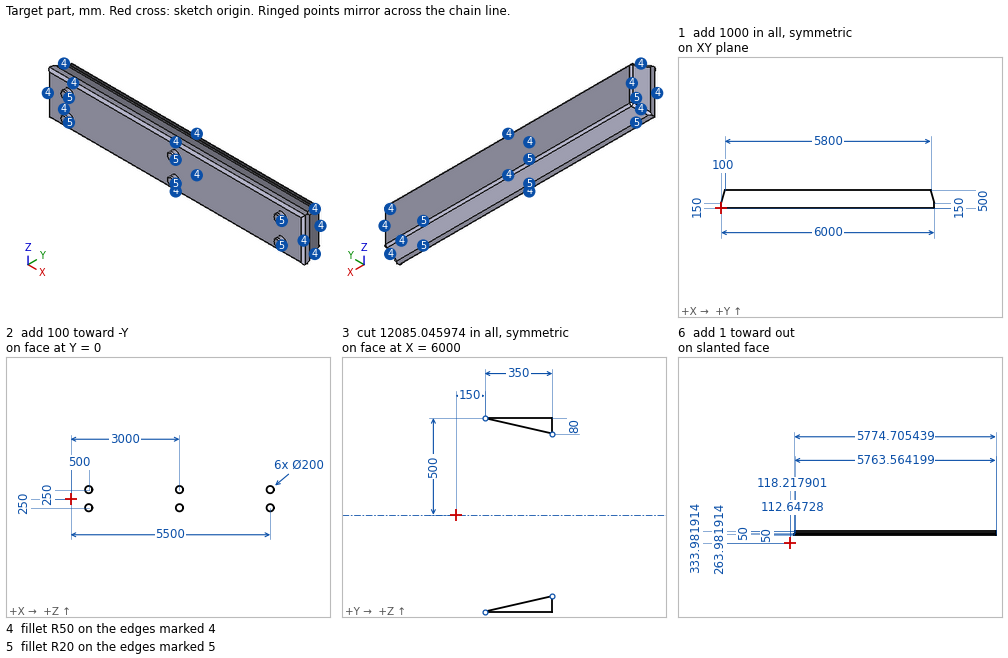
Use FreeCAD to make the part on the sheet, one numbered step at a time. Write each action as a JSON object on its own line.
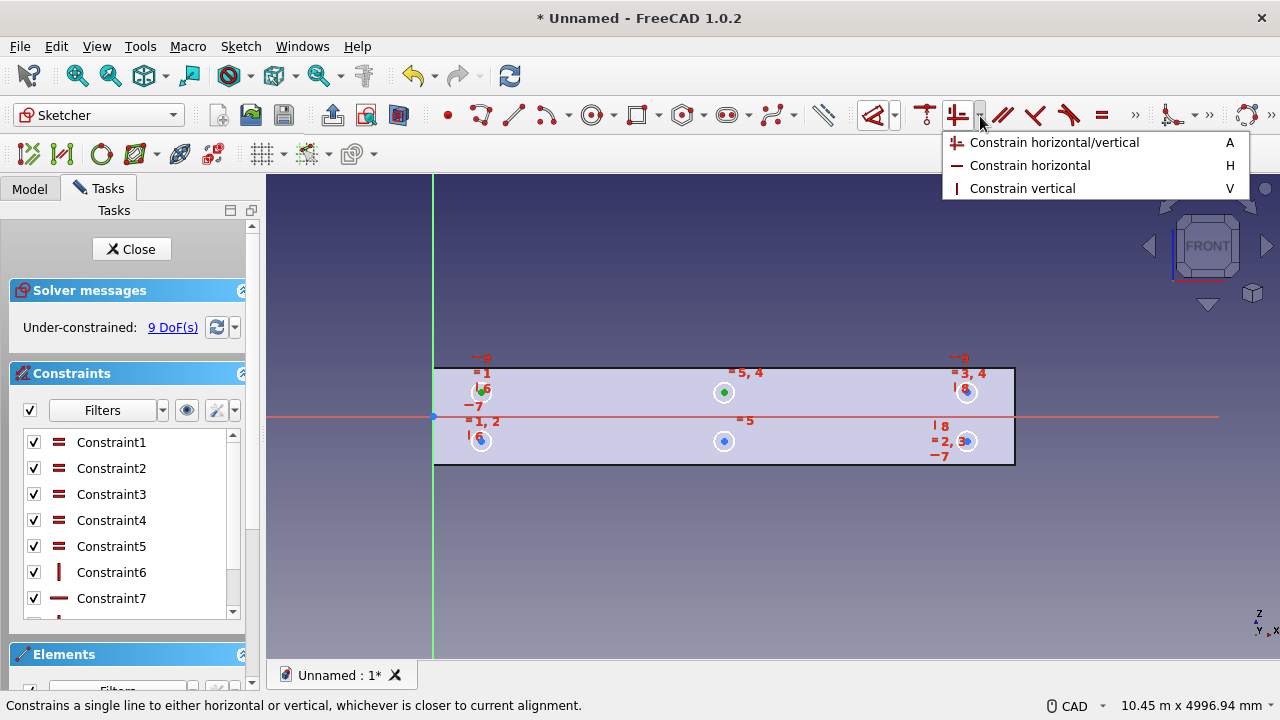
{"action": "left_click", "coordinate": [1096, 166]}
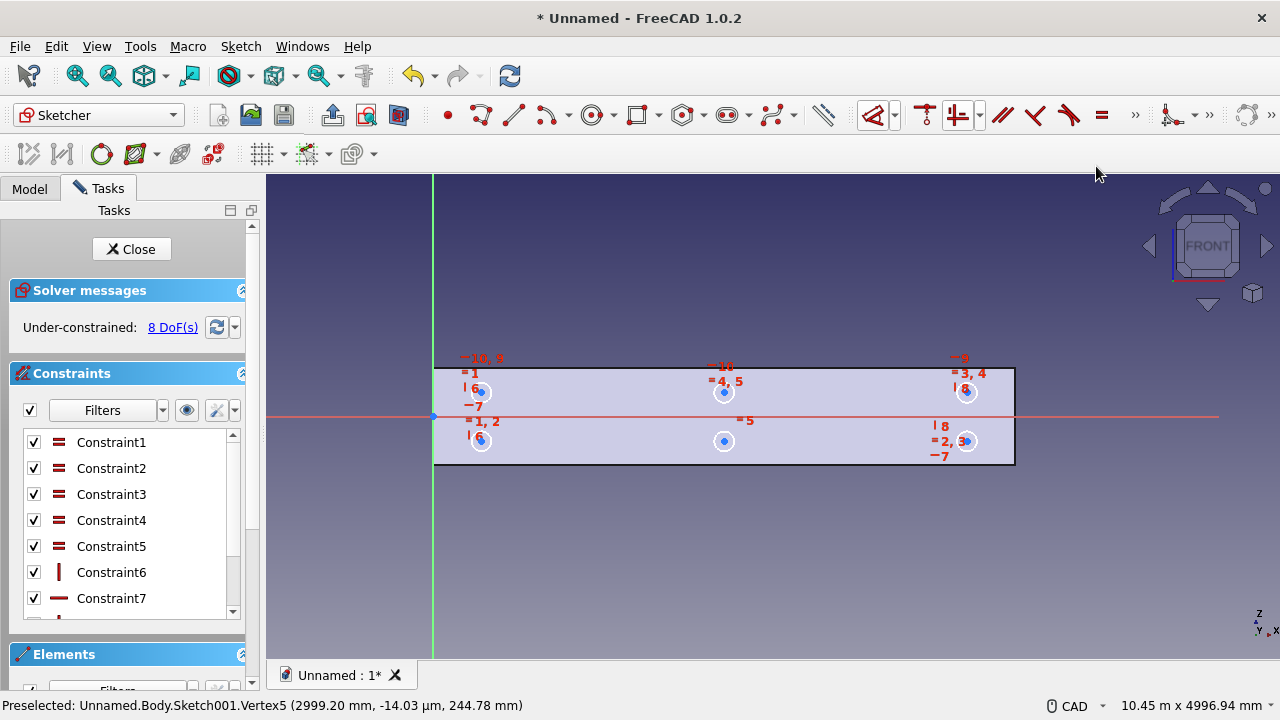
{"action": "left_click", "coordinate": [724, 393]}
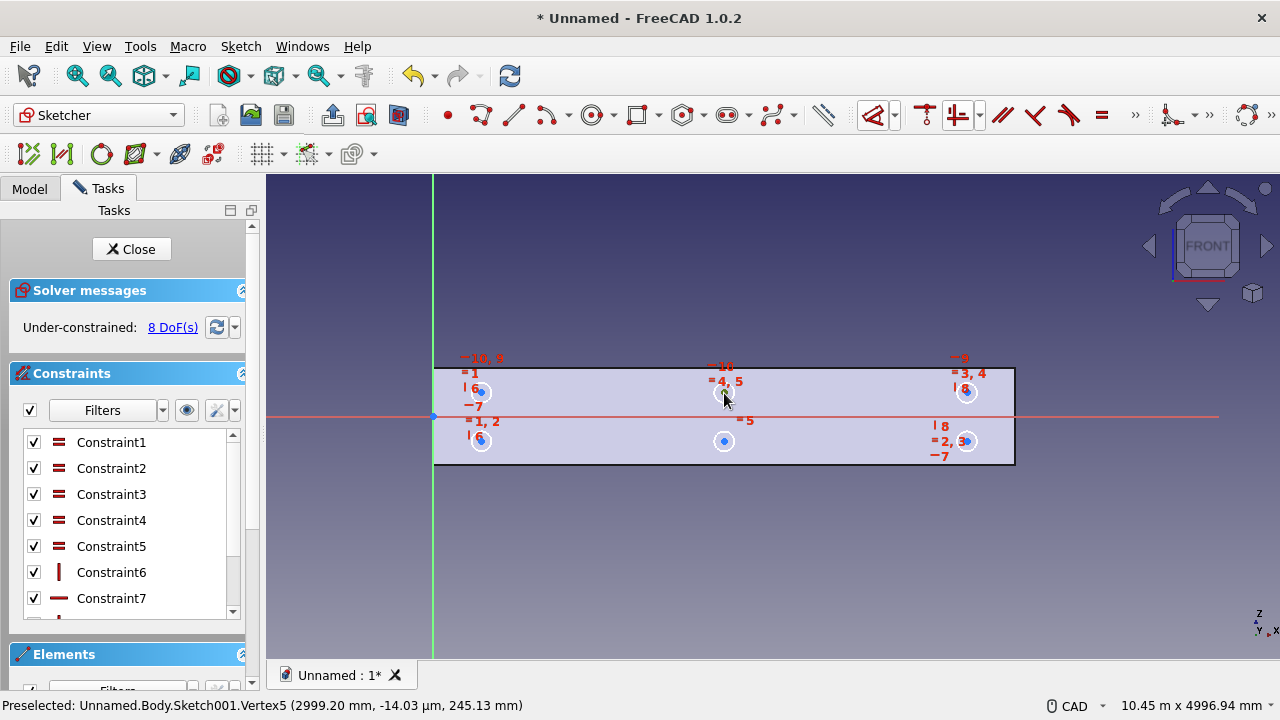
{"action": "left_click", "coordinate": [724, 441]}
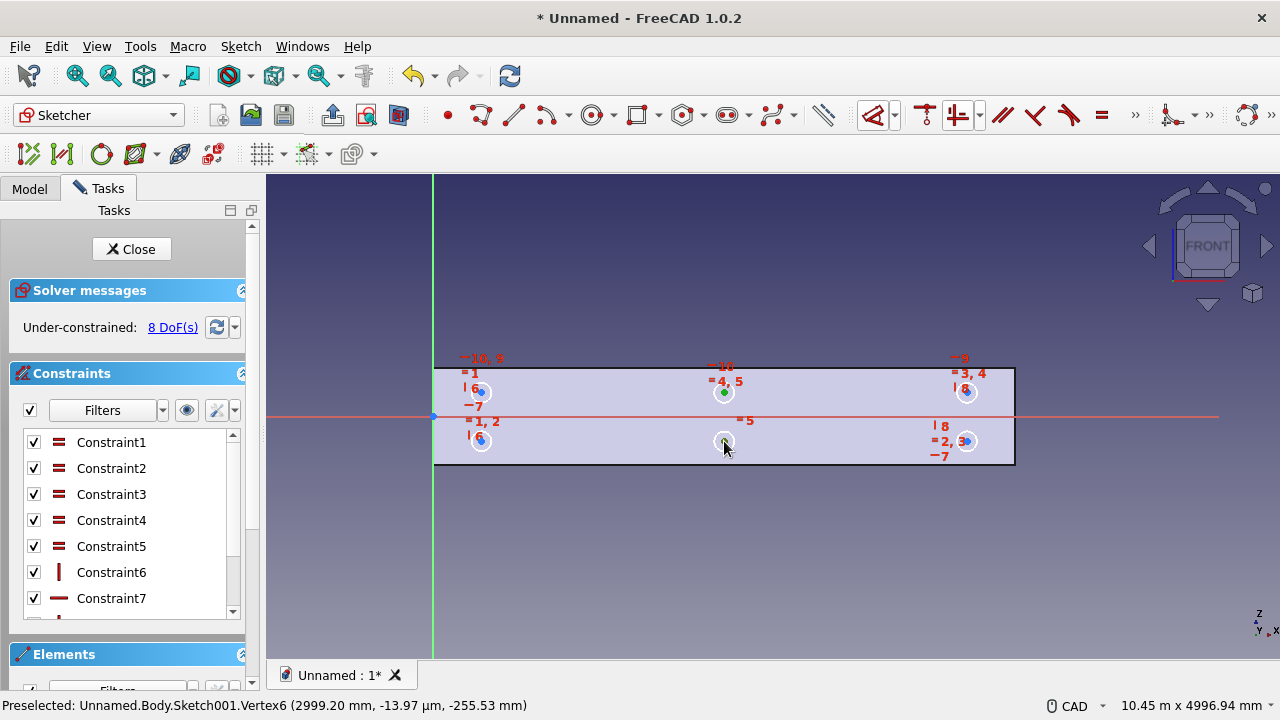
{"action": "key", "text": "v"}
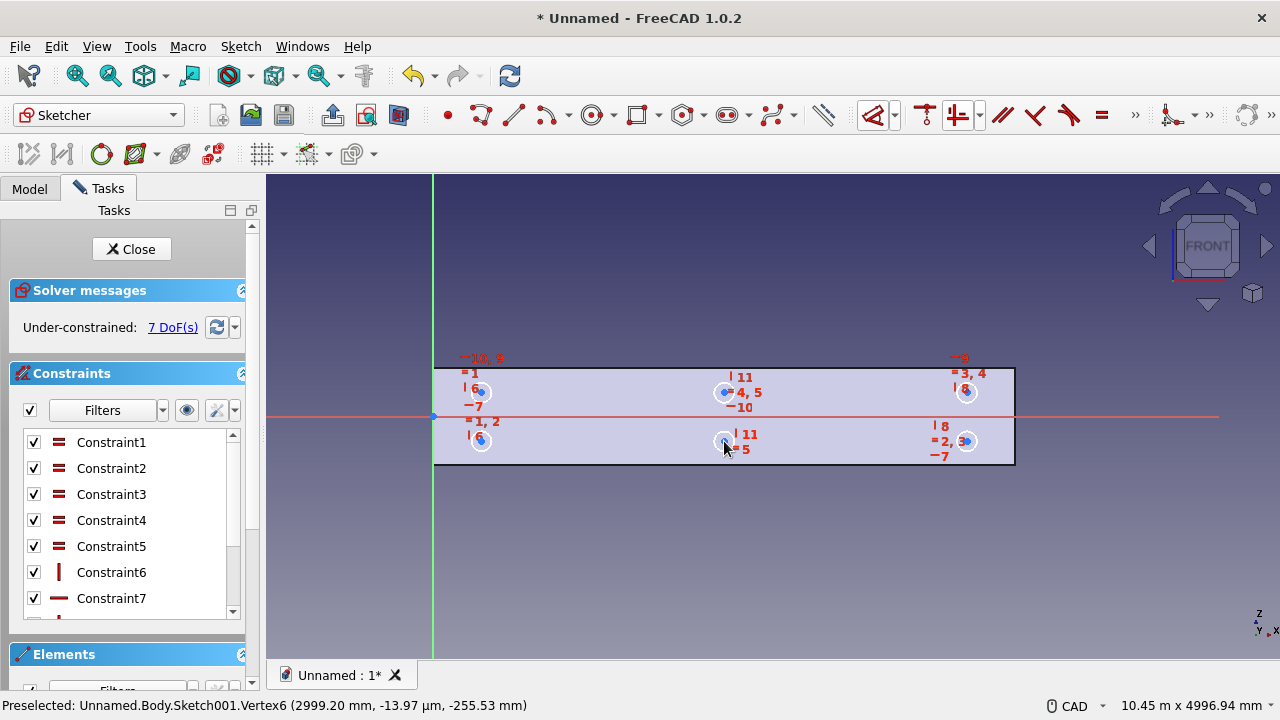
{"action": "left_click", "coordinate": [481, 441]}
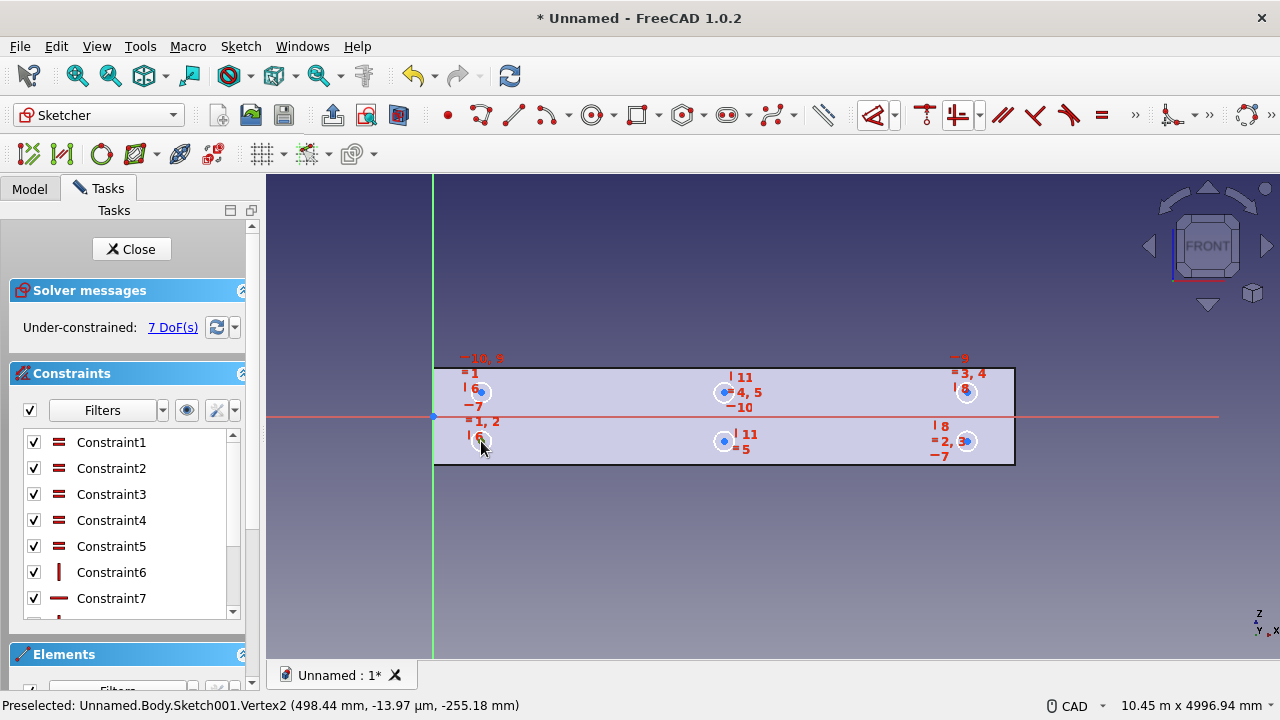
{"action": "left_click", "coordinate": [724, 441]}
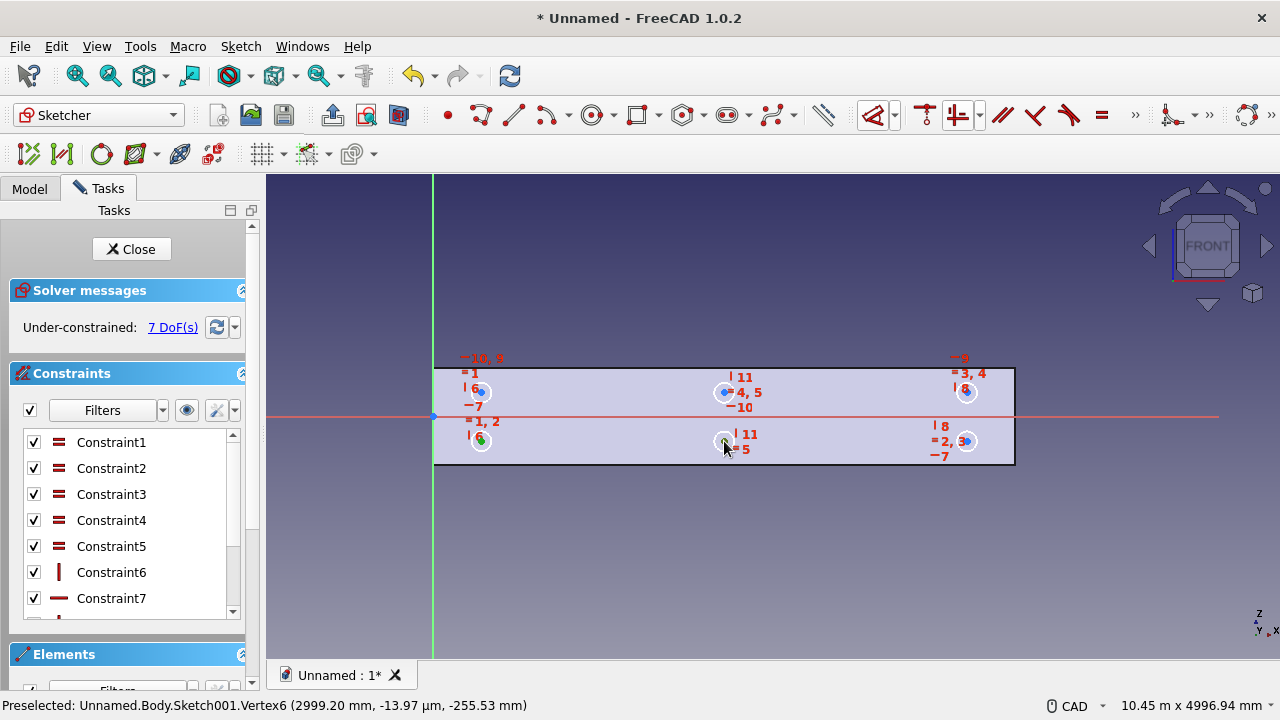
{"action": "key", "text": "h"}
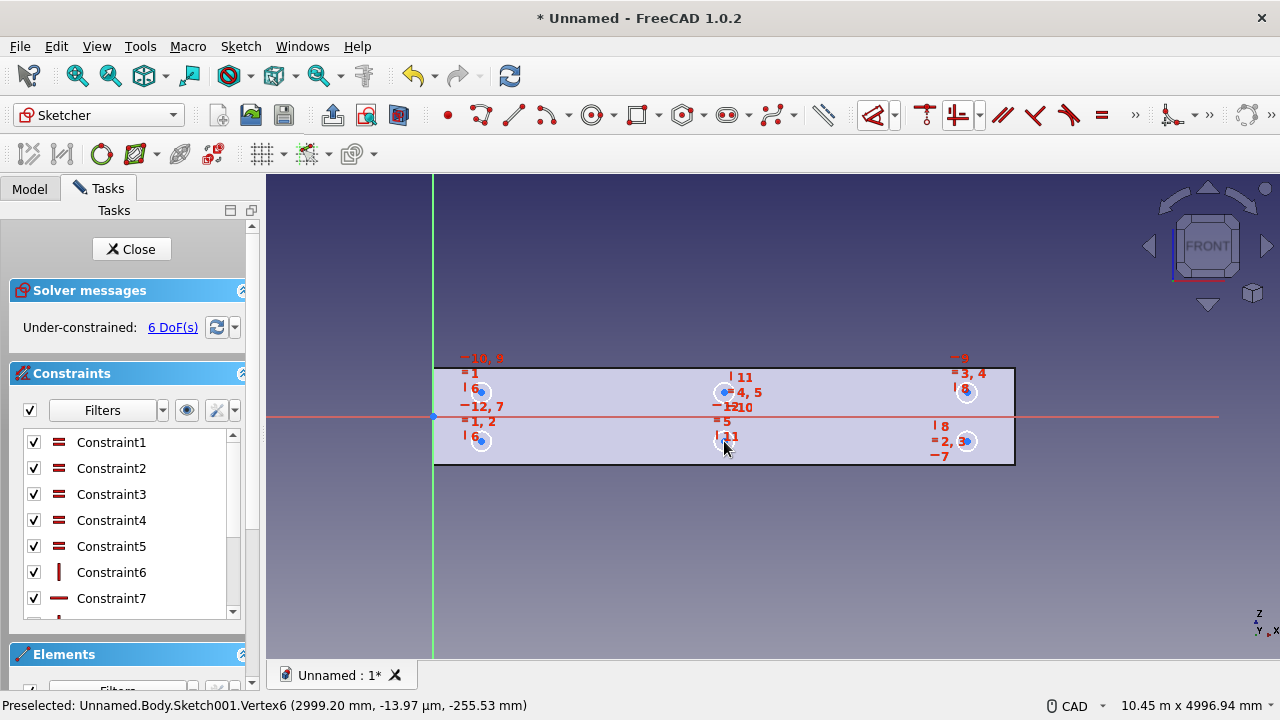
{"action": "scroll", "coordinate": [488, 386], "scroll_direction": "up", "scroll_amount": 4}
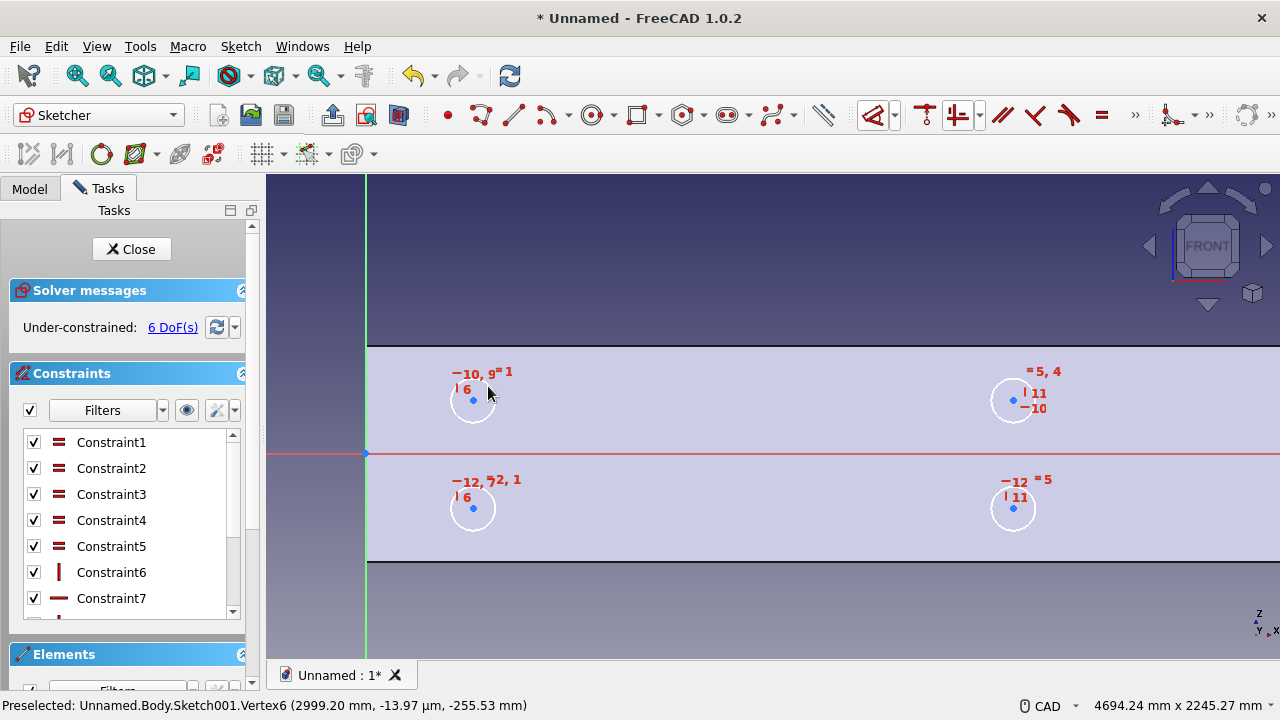
{"action": "left_click", "coordinate": [458, 416]}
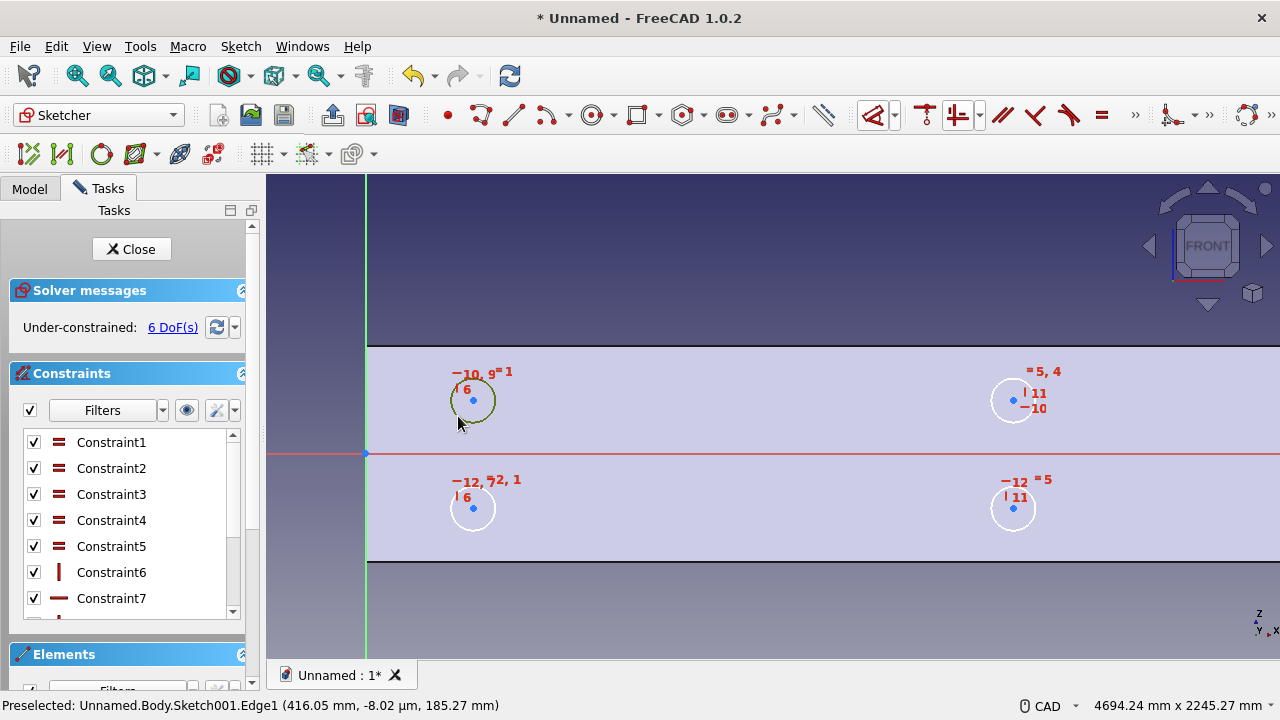
{"action": "key", "text": "k o"}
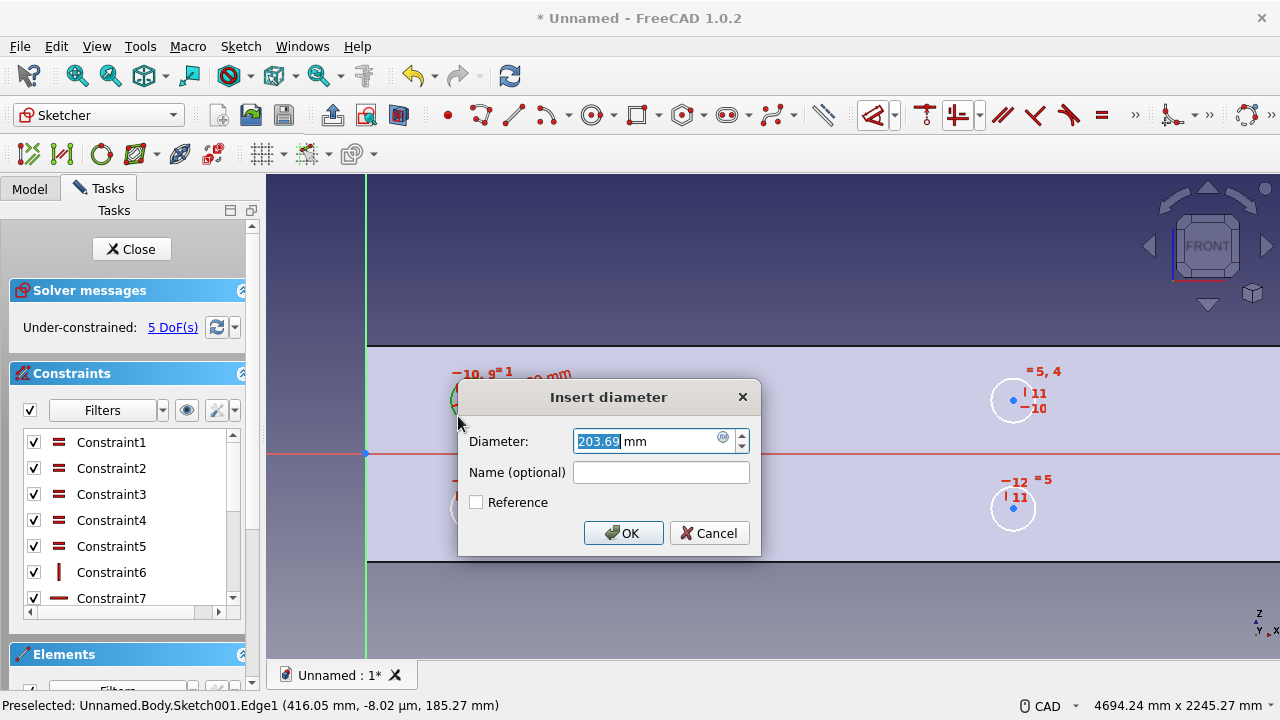
{"action": "type", "text": "200"}
{"action": "key", "text": "Return"}